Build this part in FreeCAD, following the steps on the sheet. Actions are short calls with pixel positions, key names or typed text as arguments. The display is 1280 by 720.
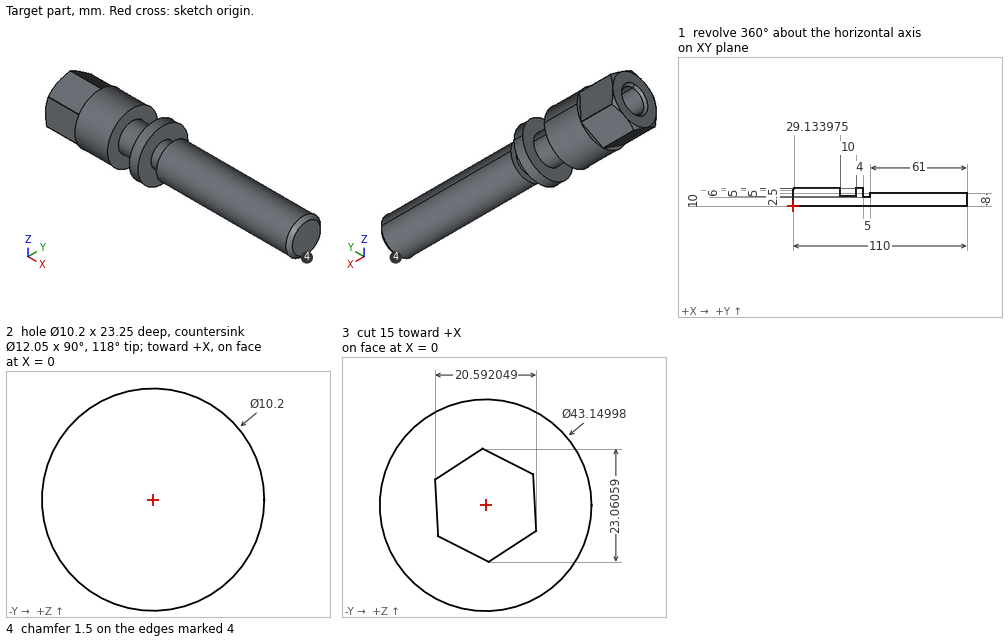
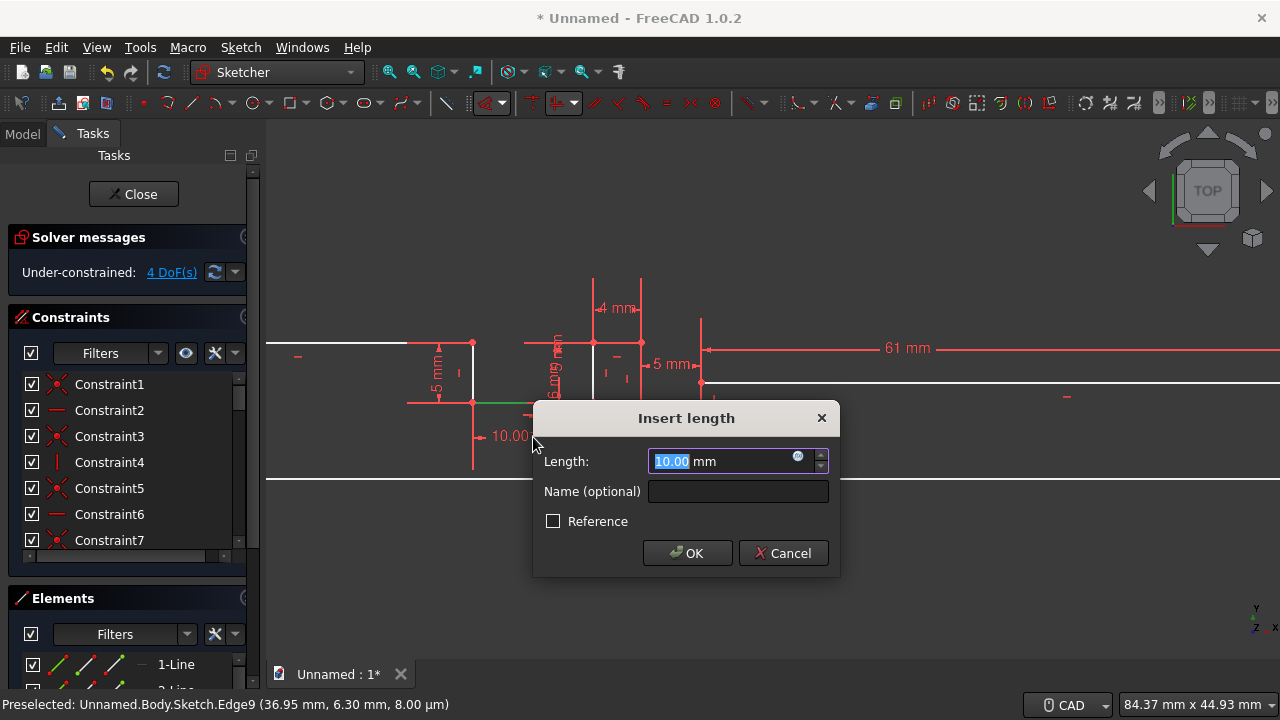
text(10)
key(Return)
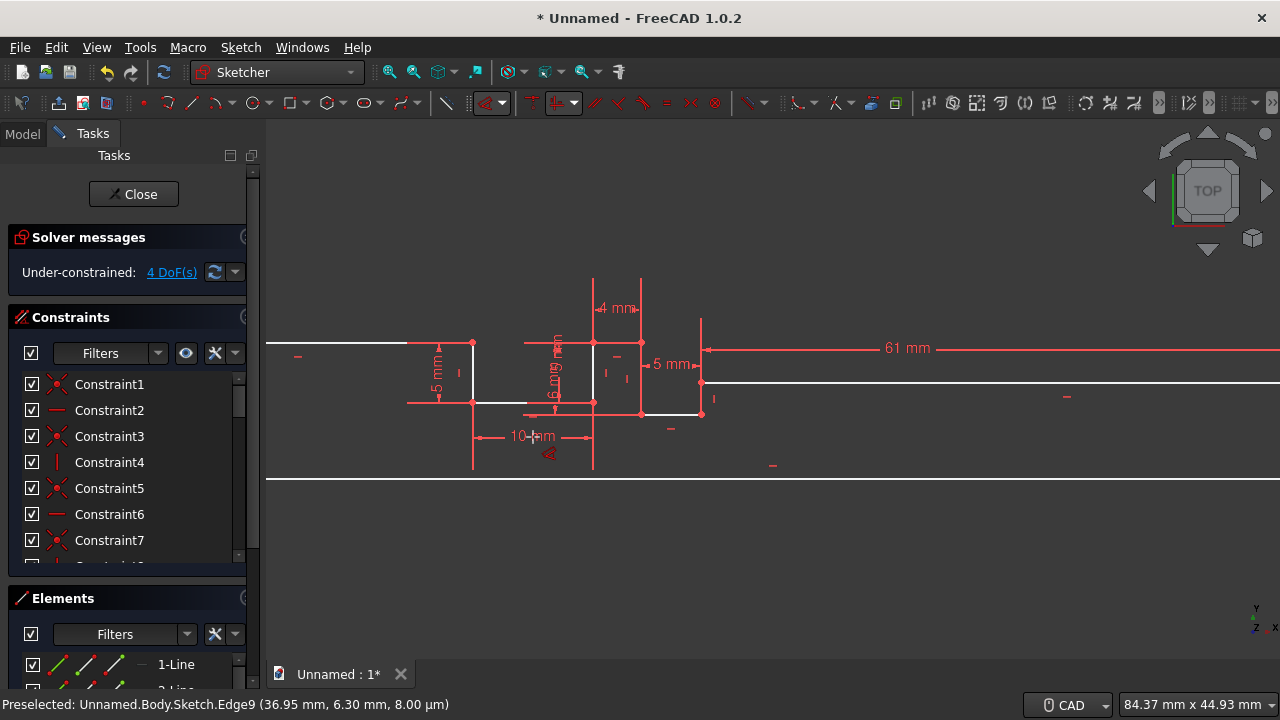
scroll(648, 372, down, 4)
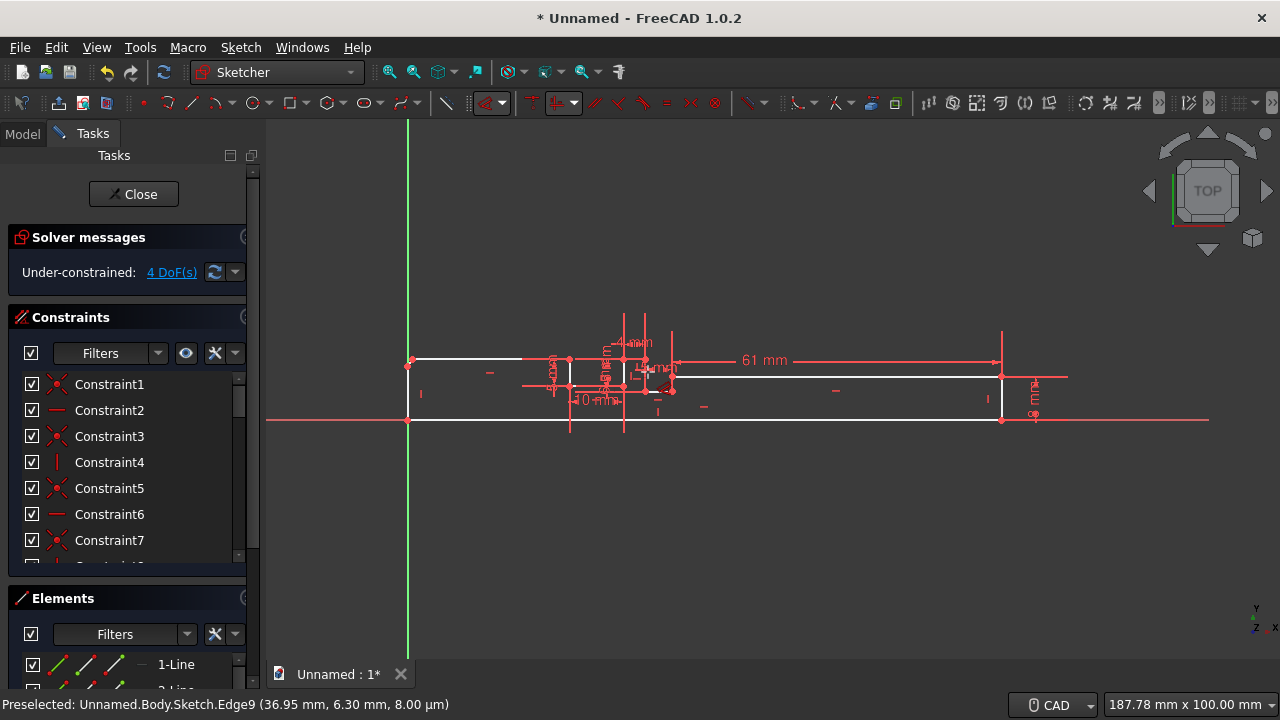
click(408, 383)
click(374, 393)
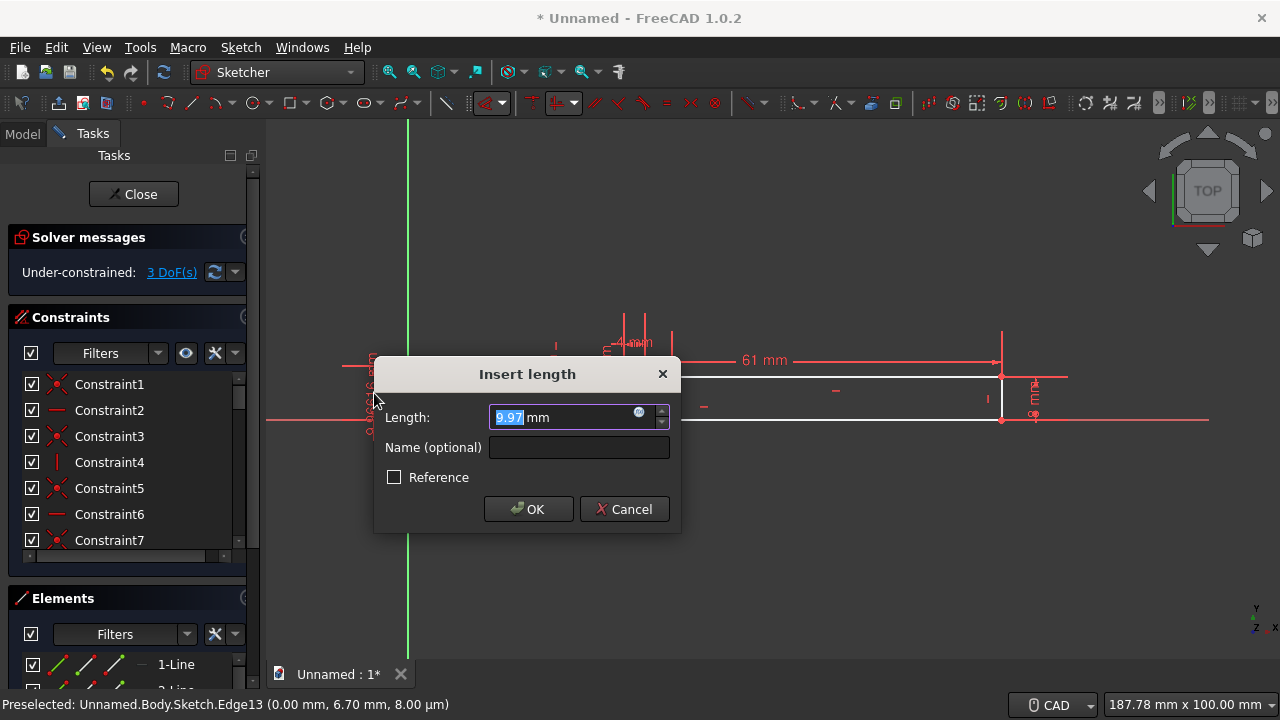
text(10)
key(Return)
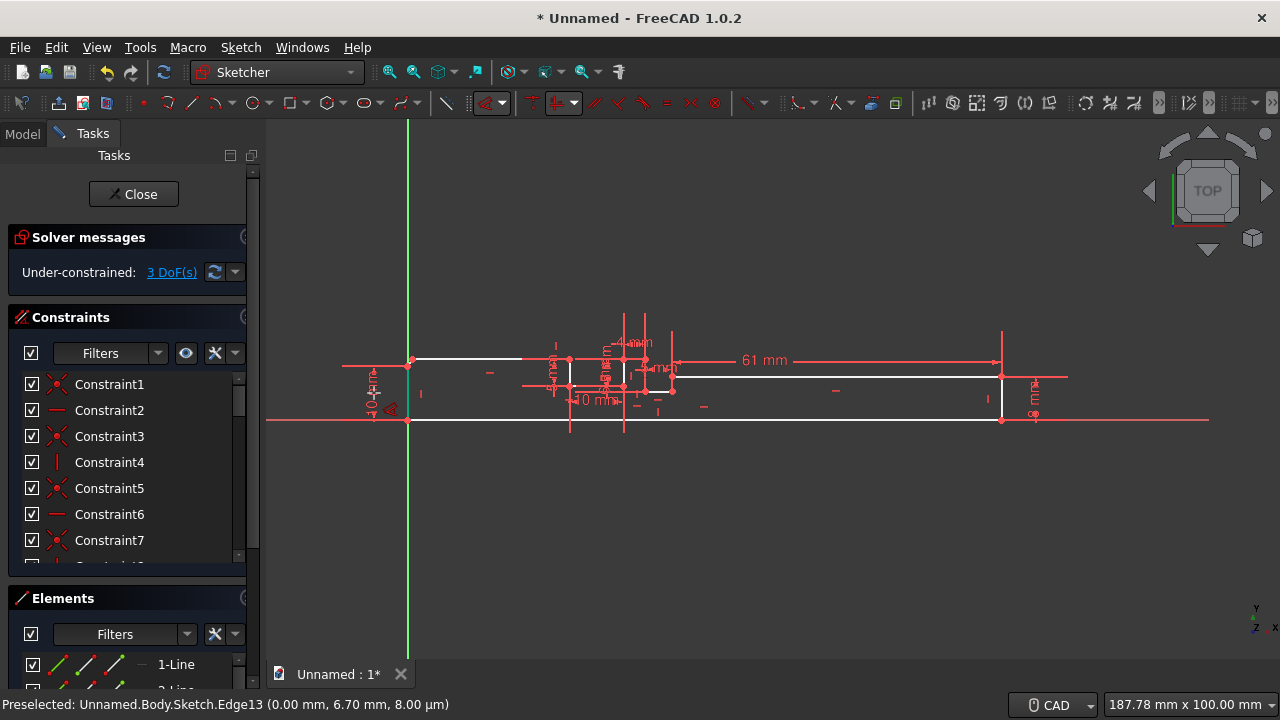
click(586, 420)
click(705, 454)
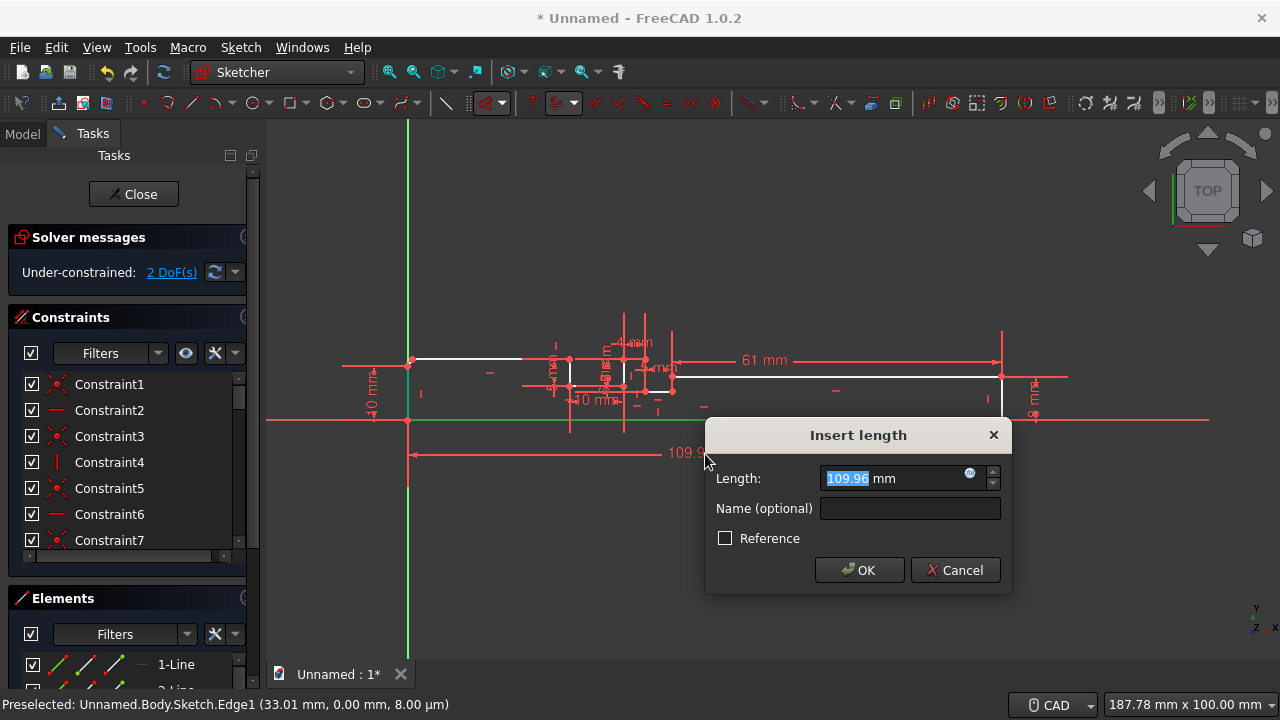
text(110)
key(Return)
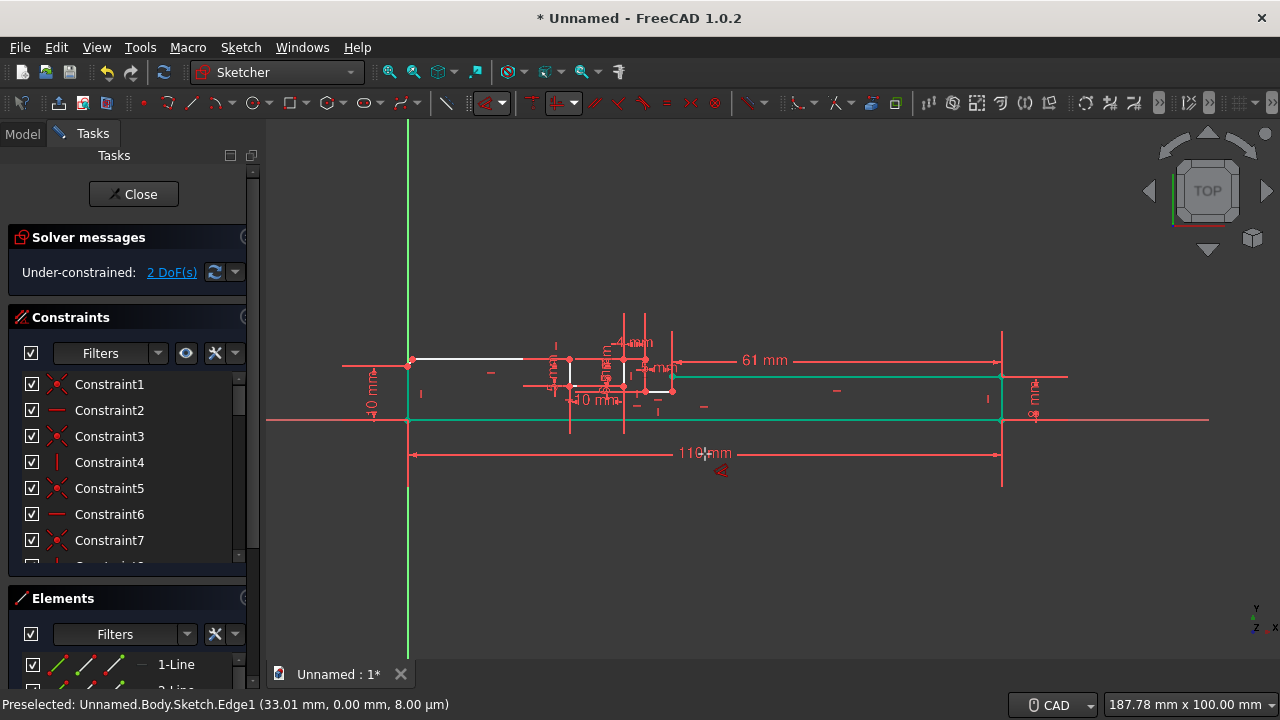
scroll(672, 384, up, 6)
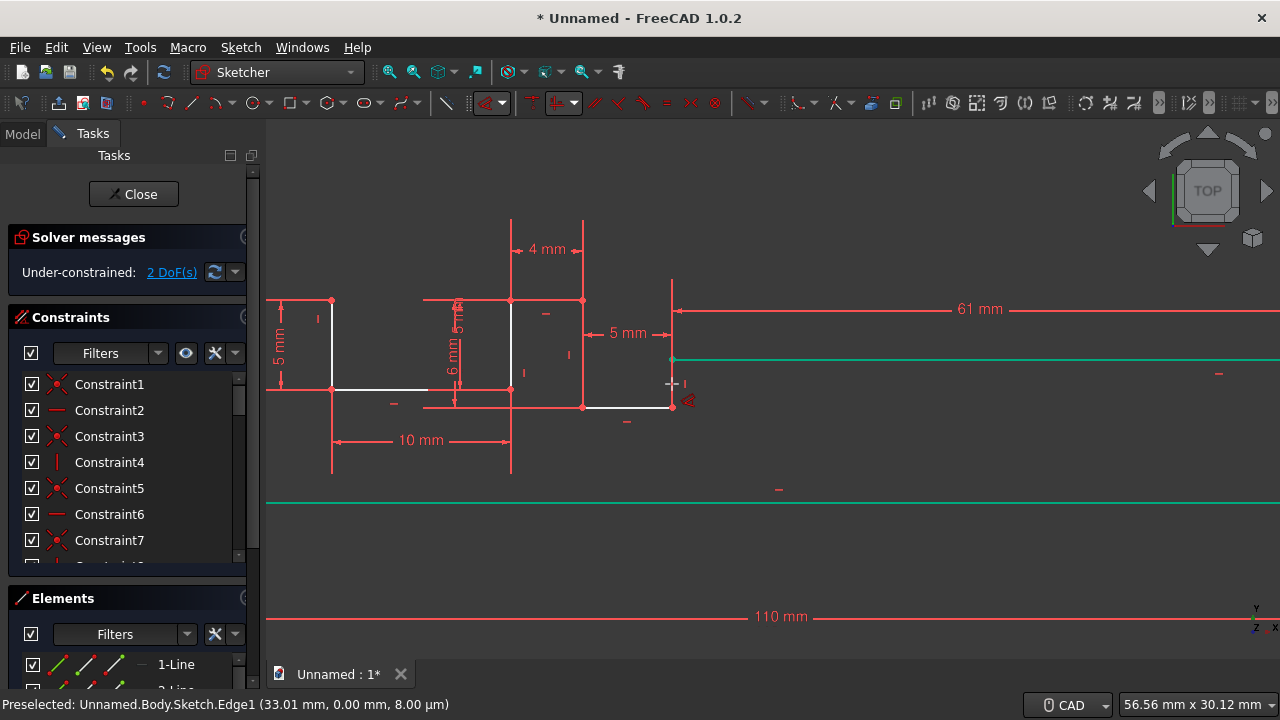
click(672, 384)
click(638, 384)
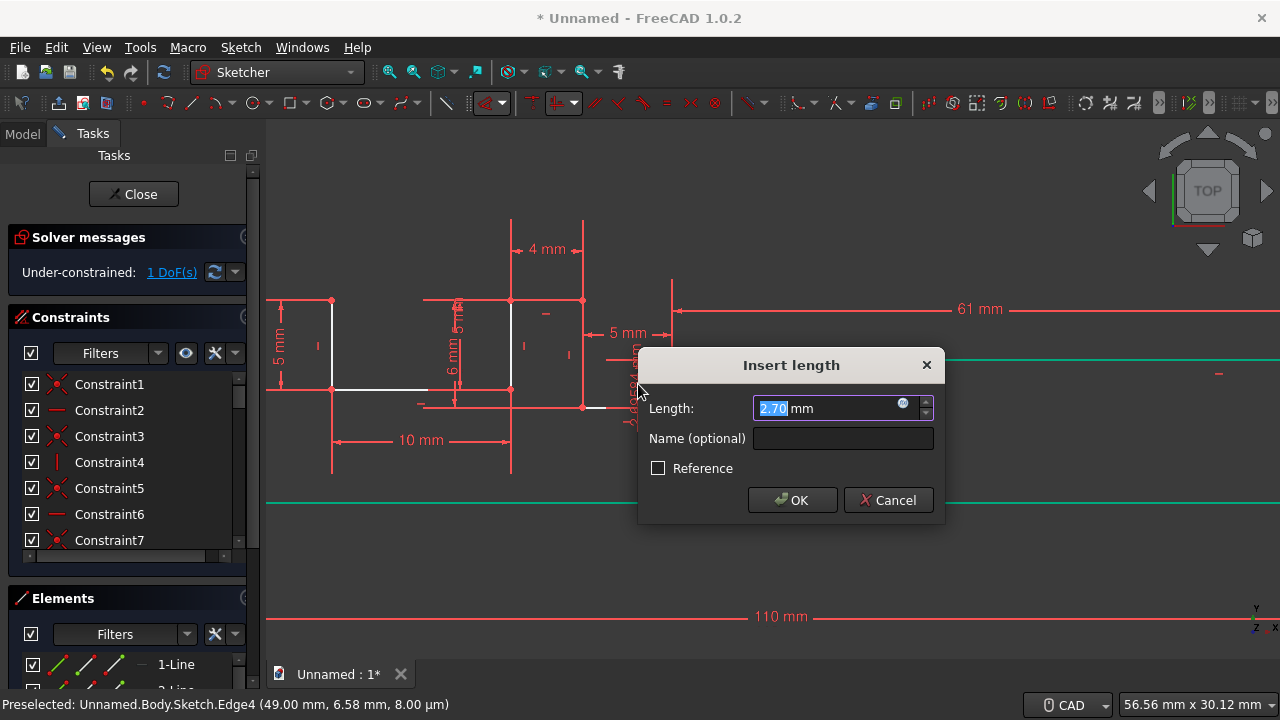
text(2.5)
key(Return)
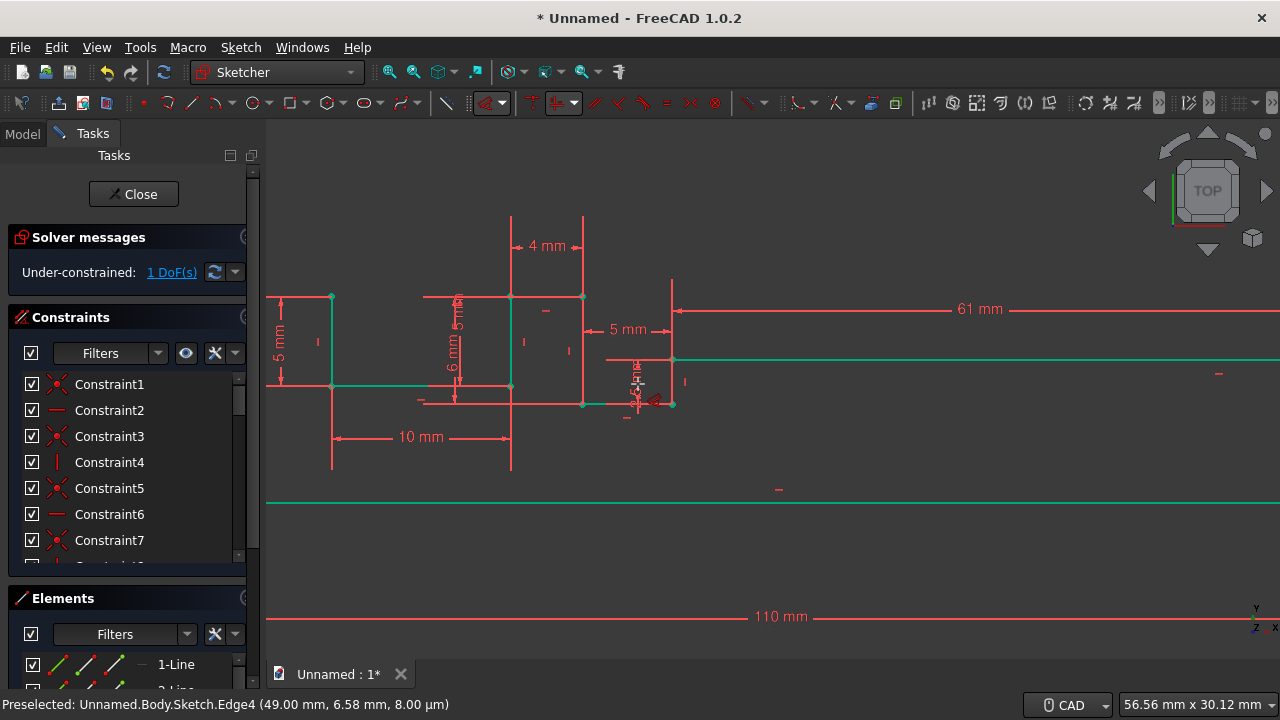
scroll(672, 384, down, 6)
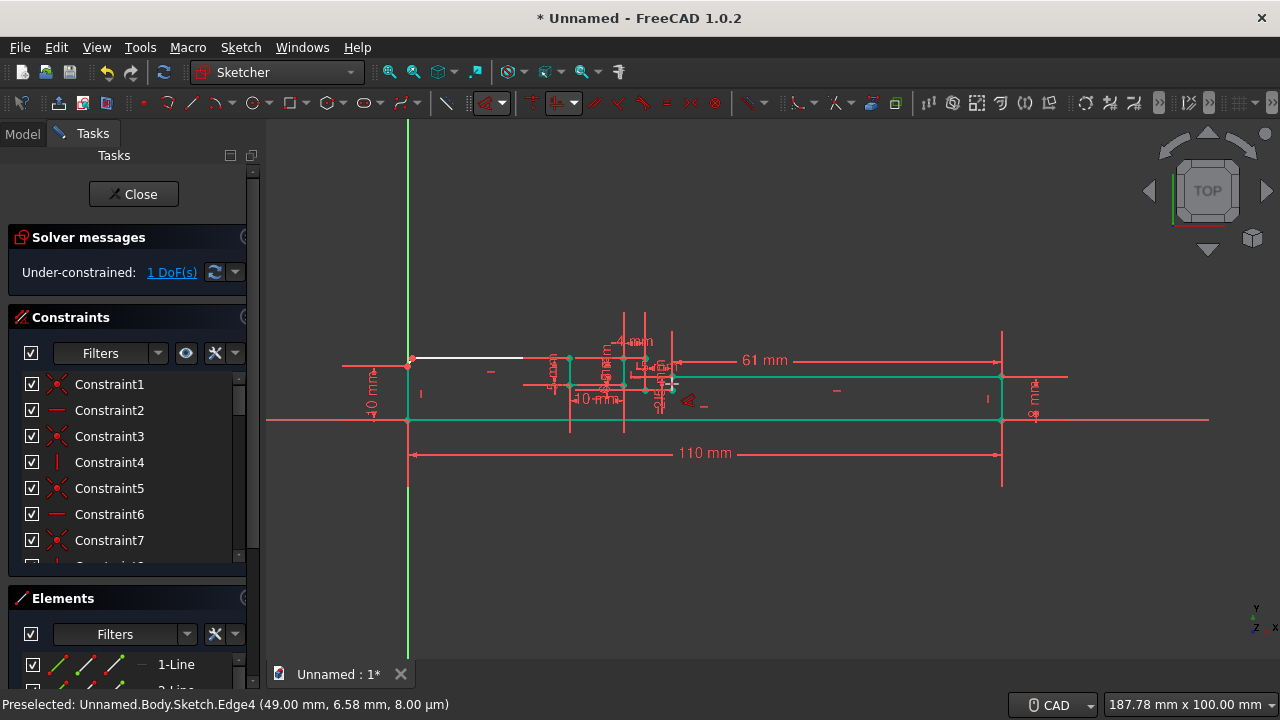
click(523, 358)
click(491, 324)